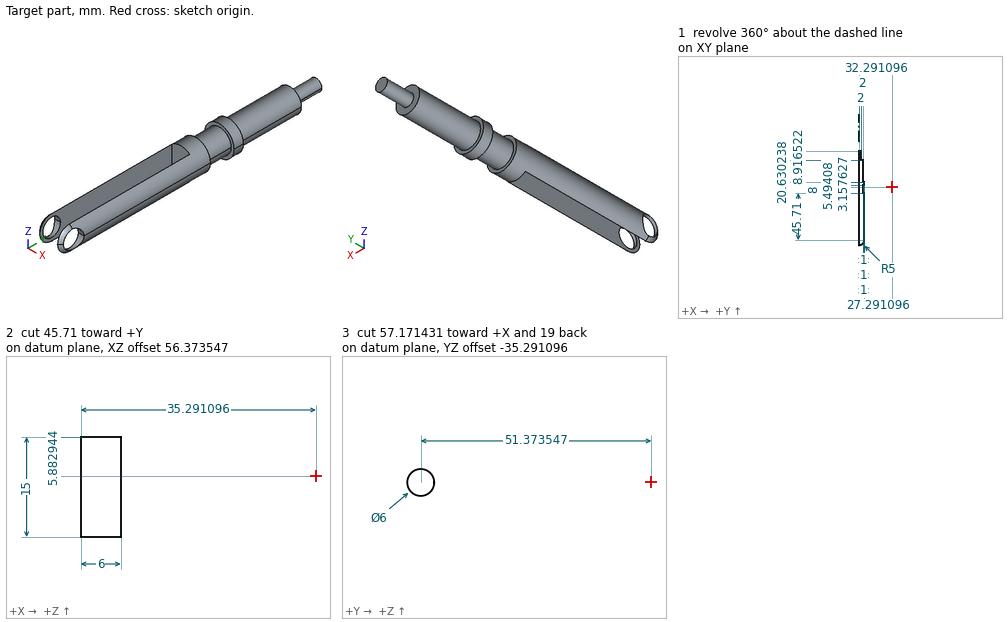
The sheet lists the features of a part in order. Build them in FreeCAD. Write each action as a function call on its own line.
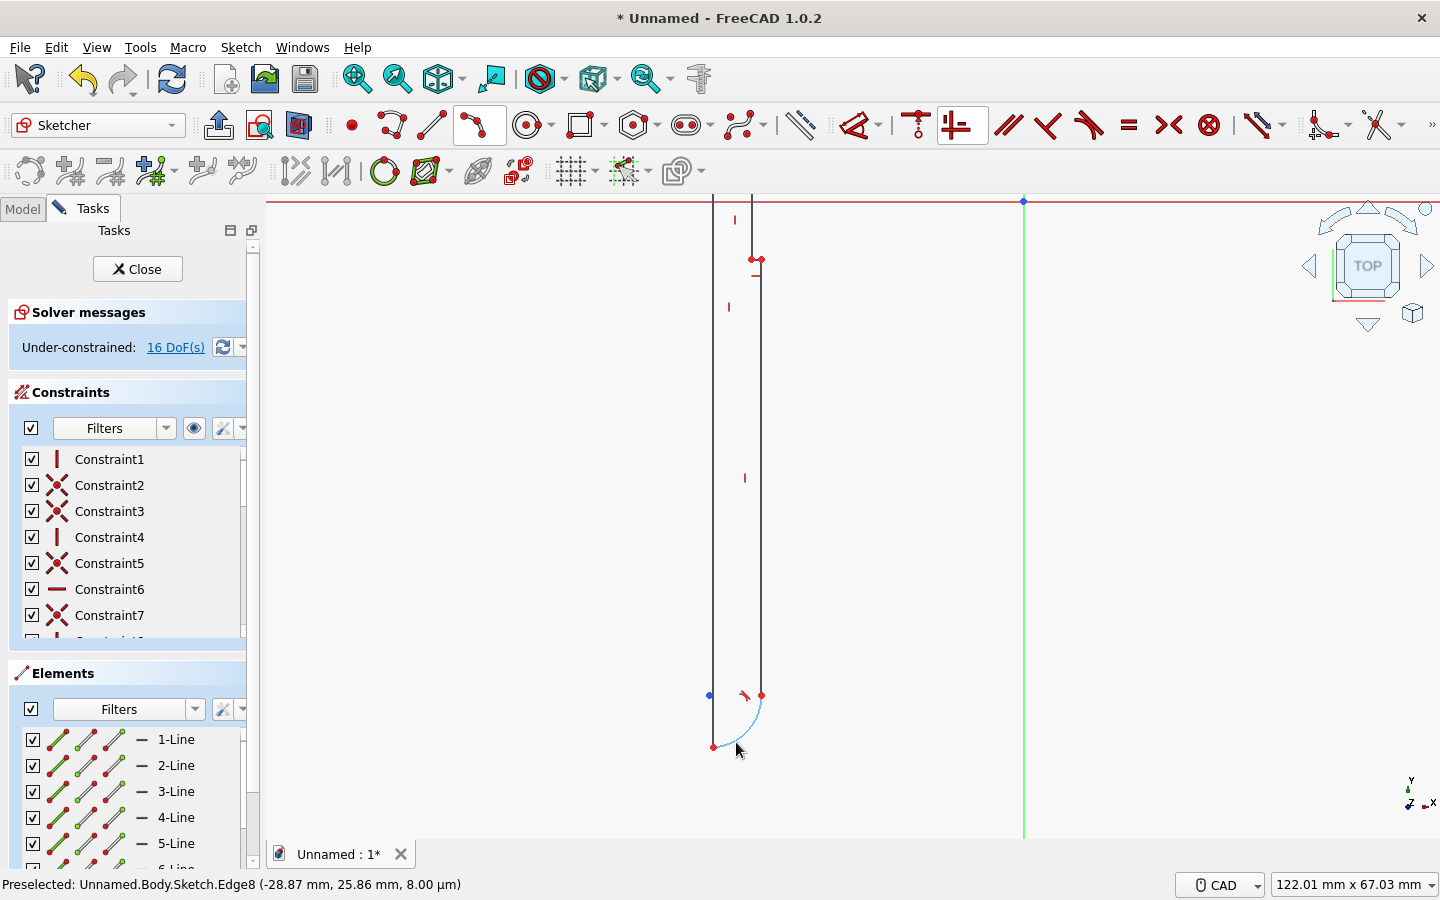
click(735, 741)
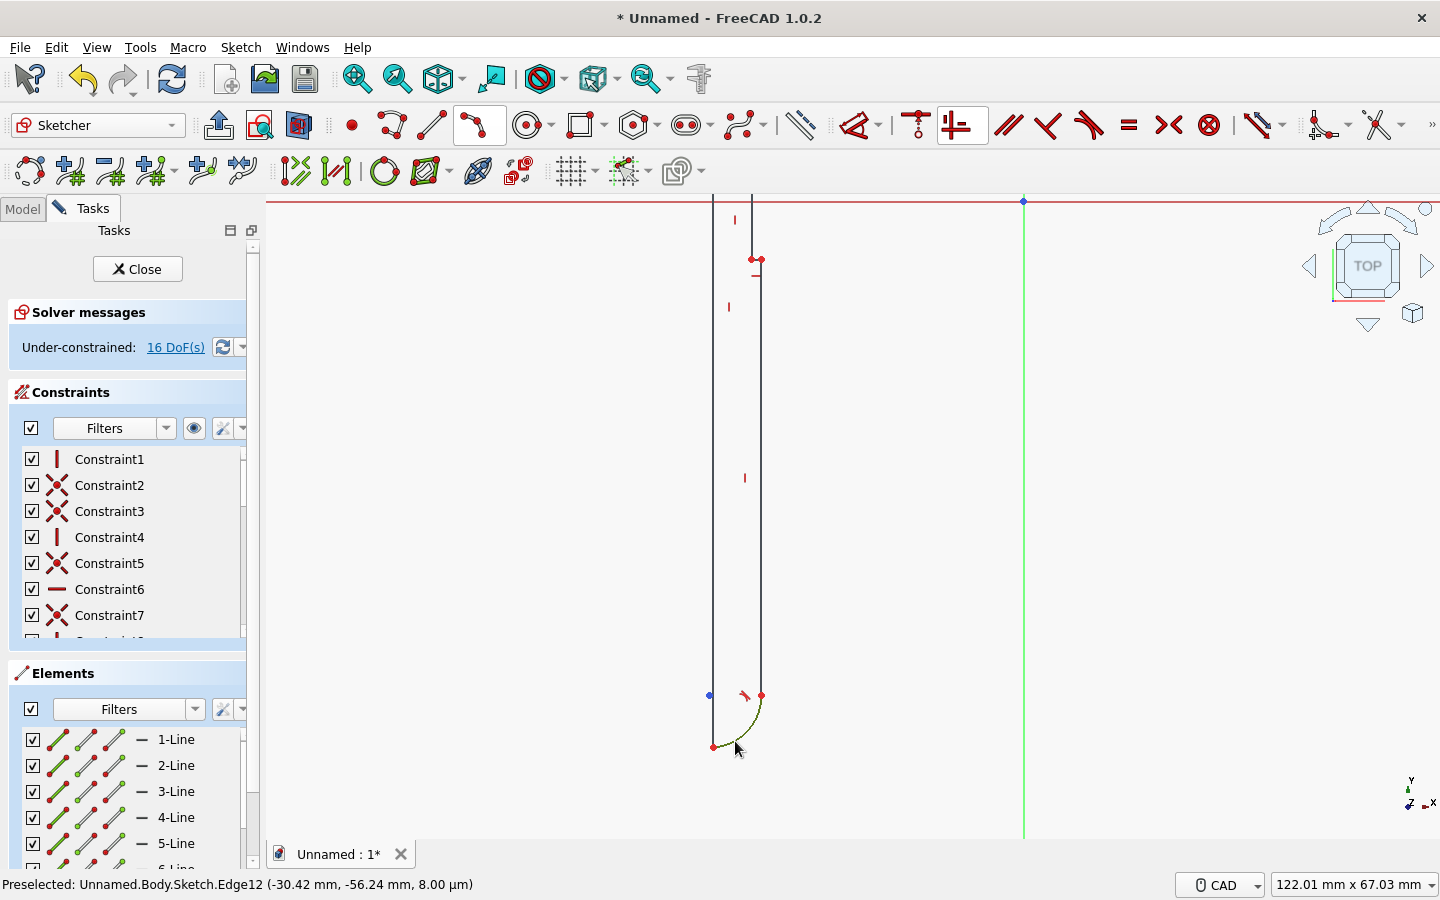
key(k)
key(r)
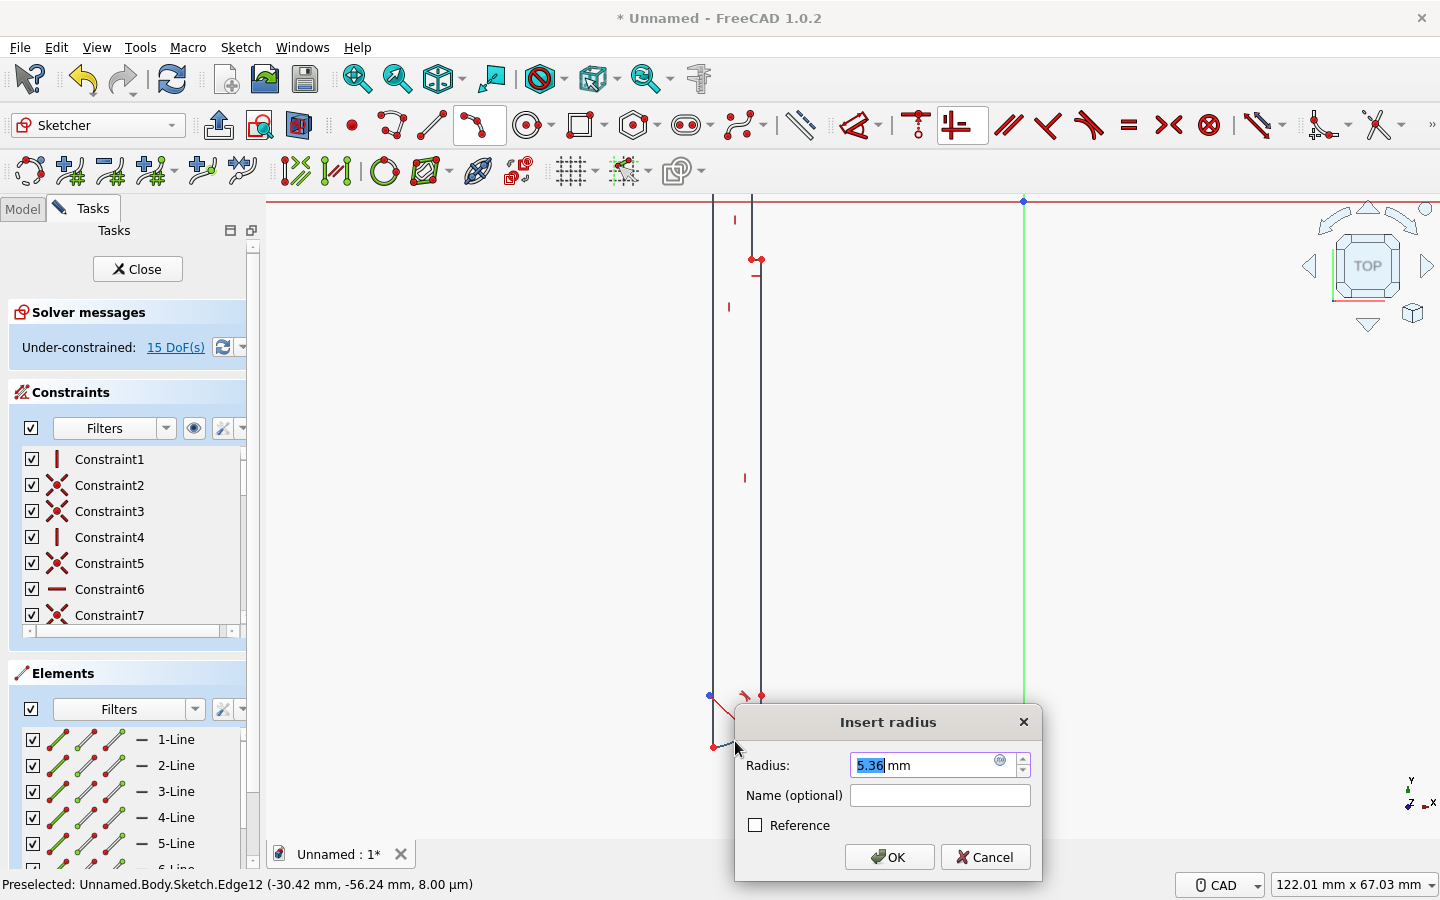
text(5)
key(Return)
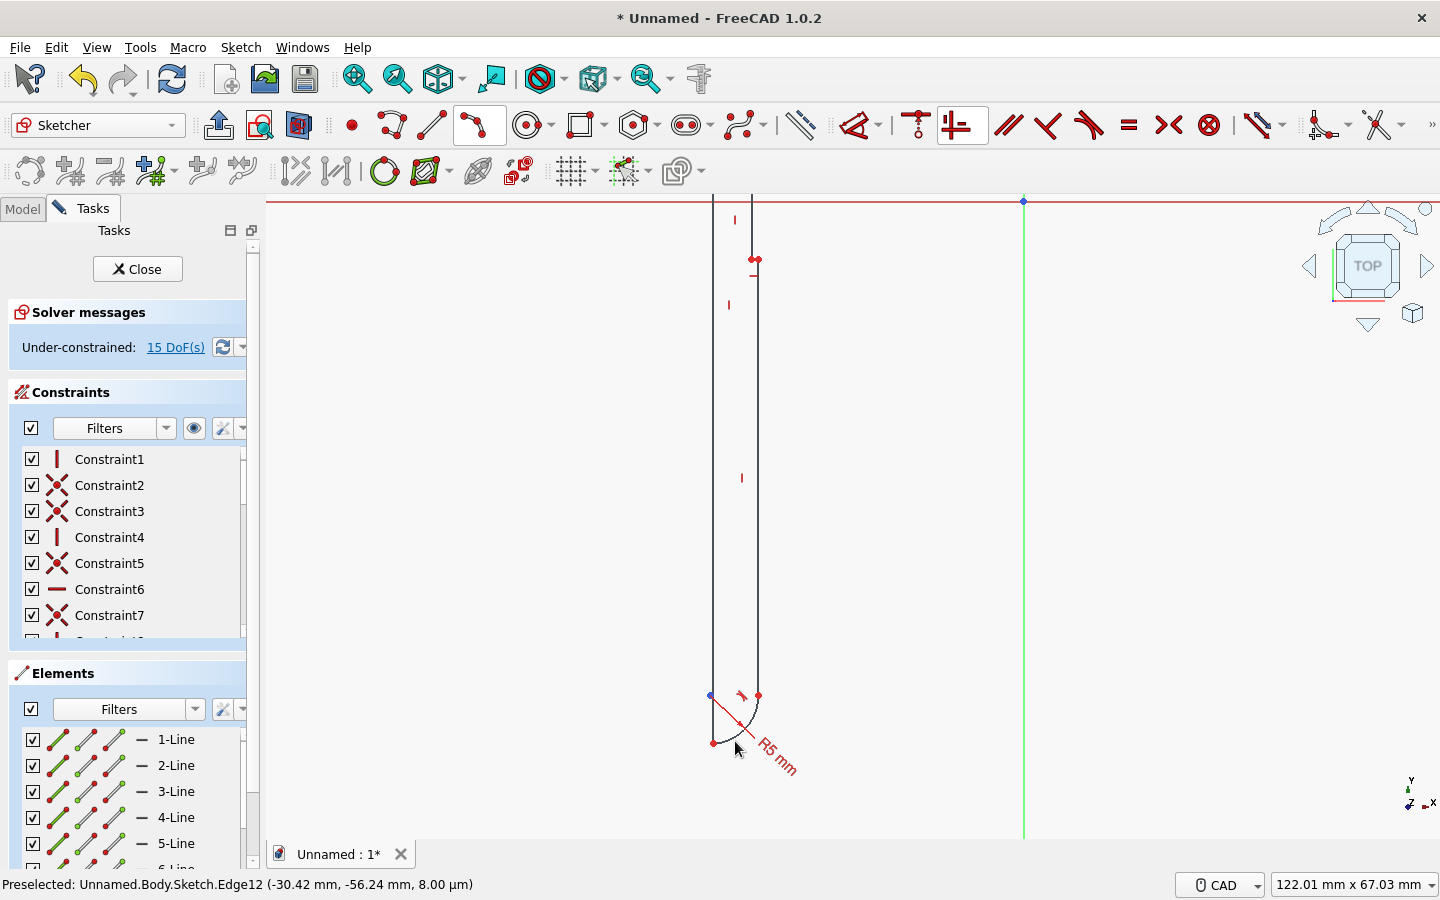
scroll(755, 260, up, 8)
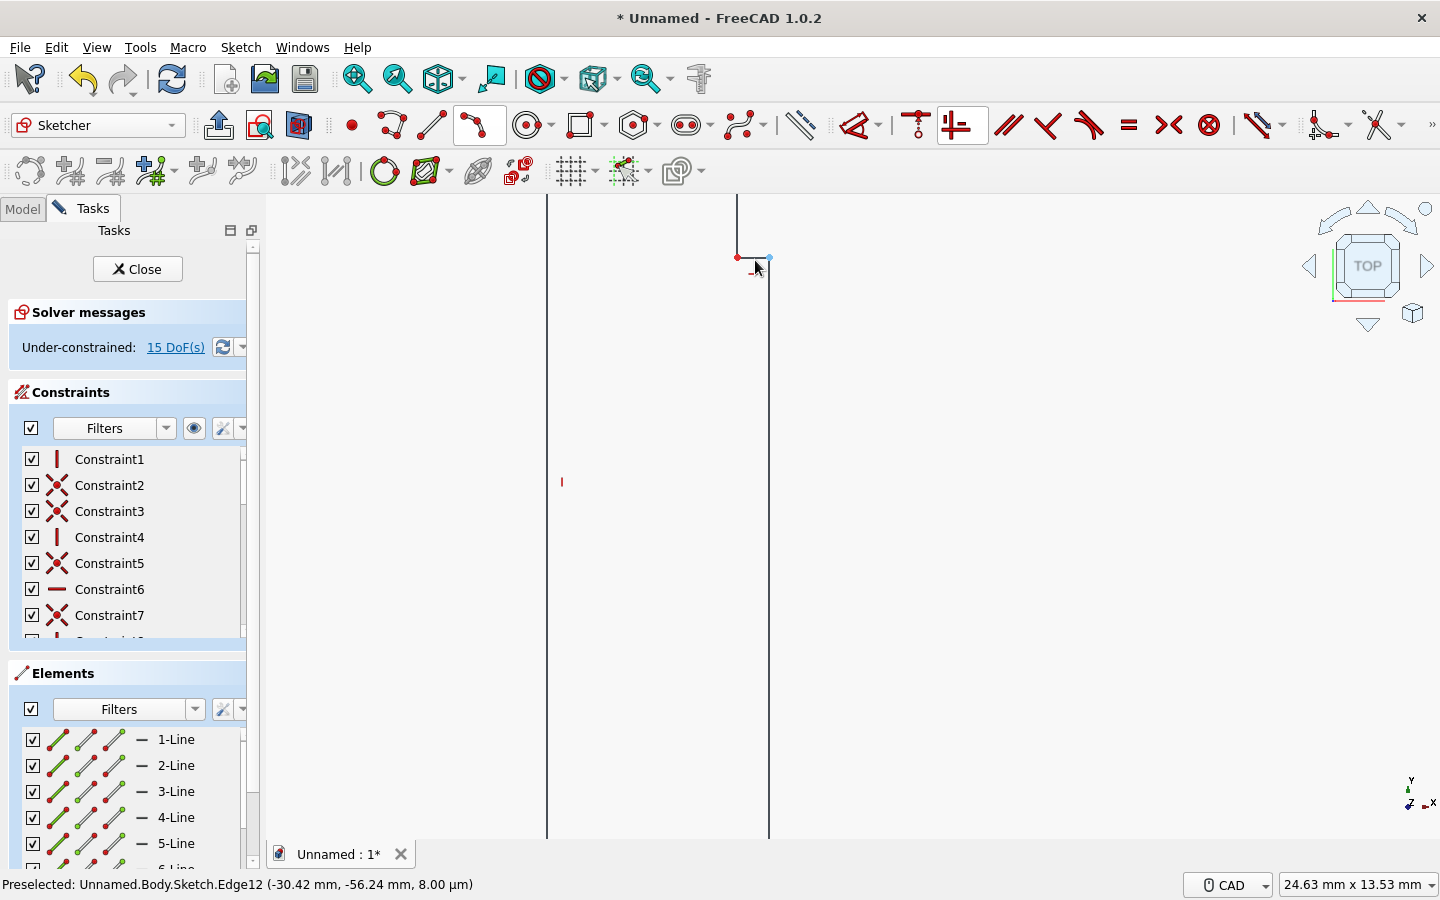
click(753, 258)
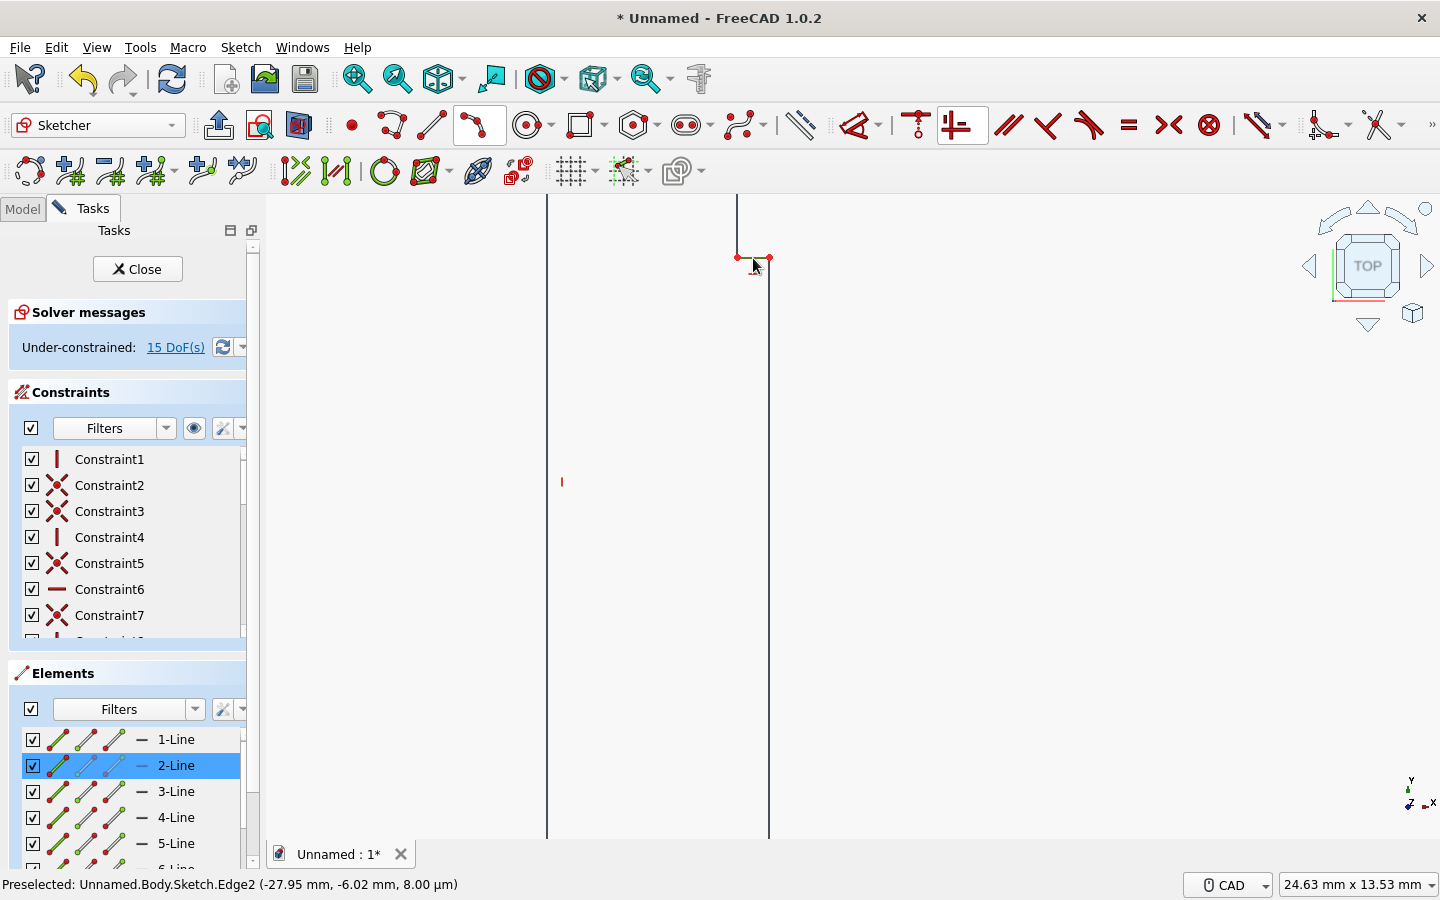
click(880, 126)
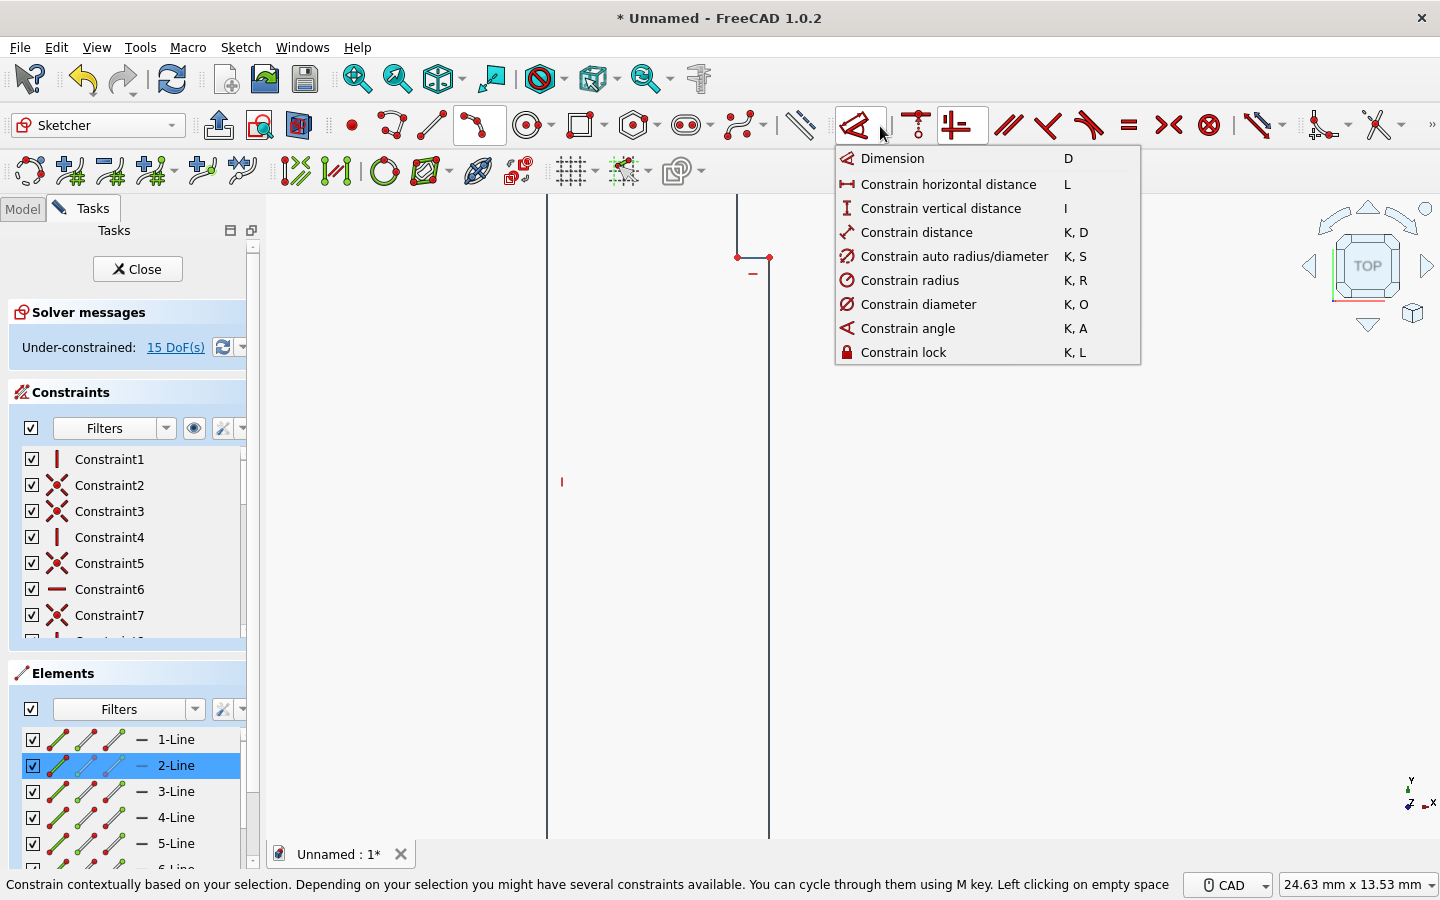
click(988, 184)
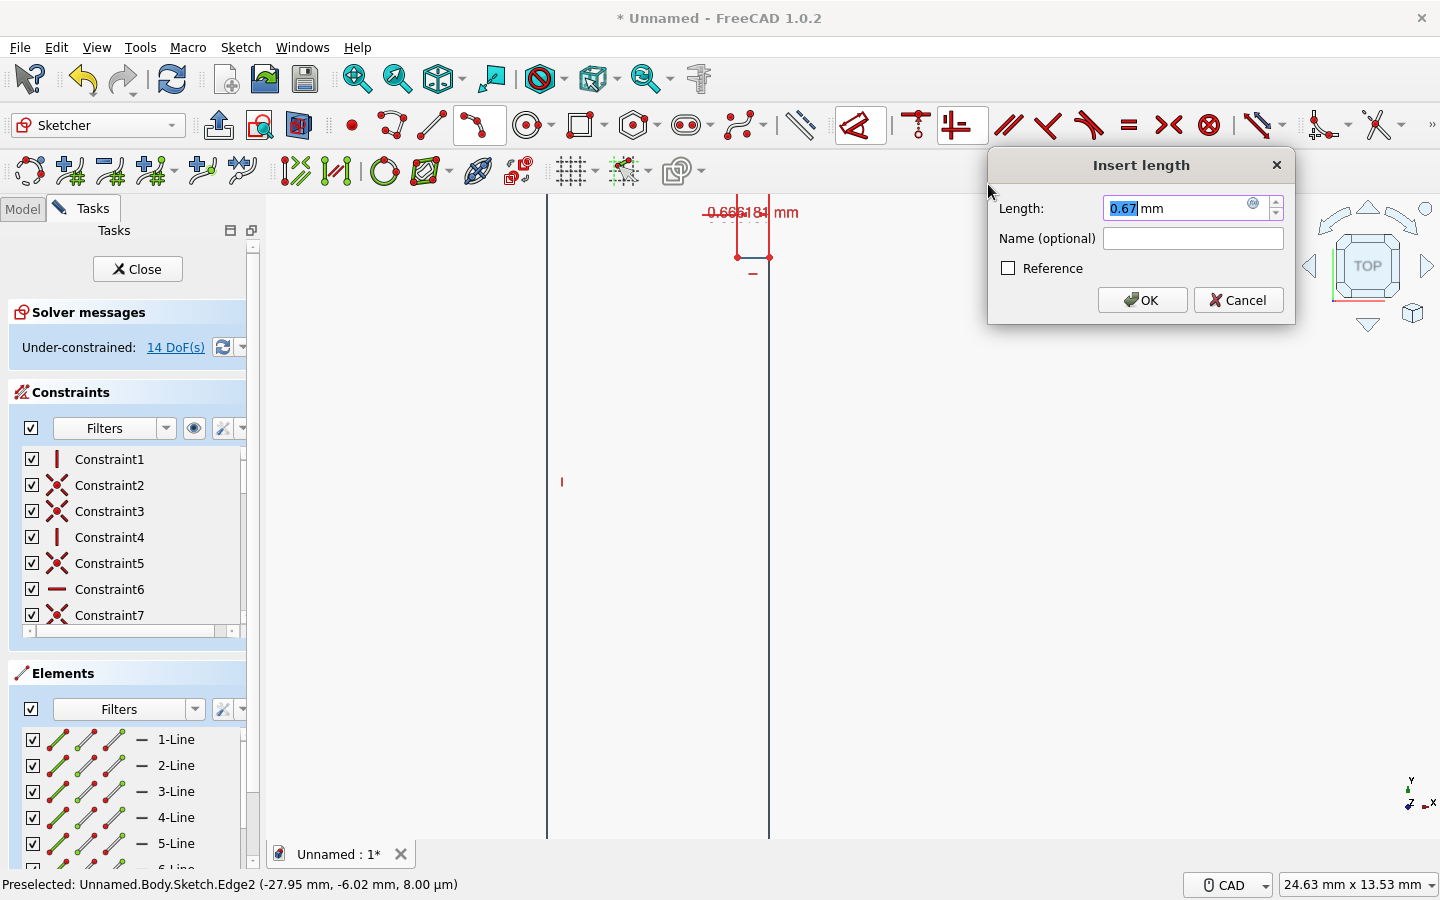
text(1)
key(Return)